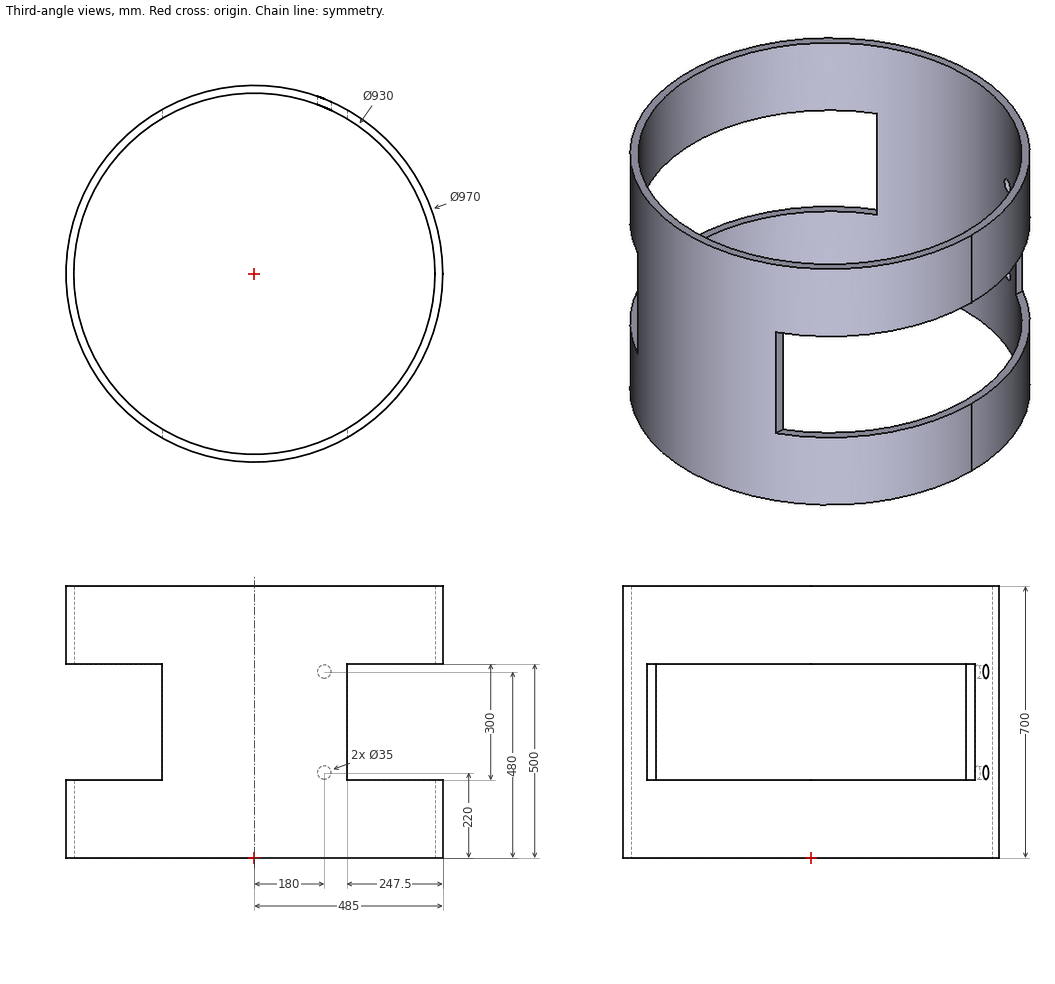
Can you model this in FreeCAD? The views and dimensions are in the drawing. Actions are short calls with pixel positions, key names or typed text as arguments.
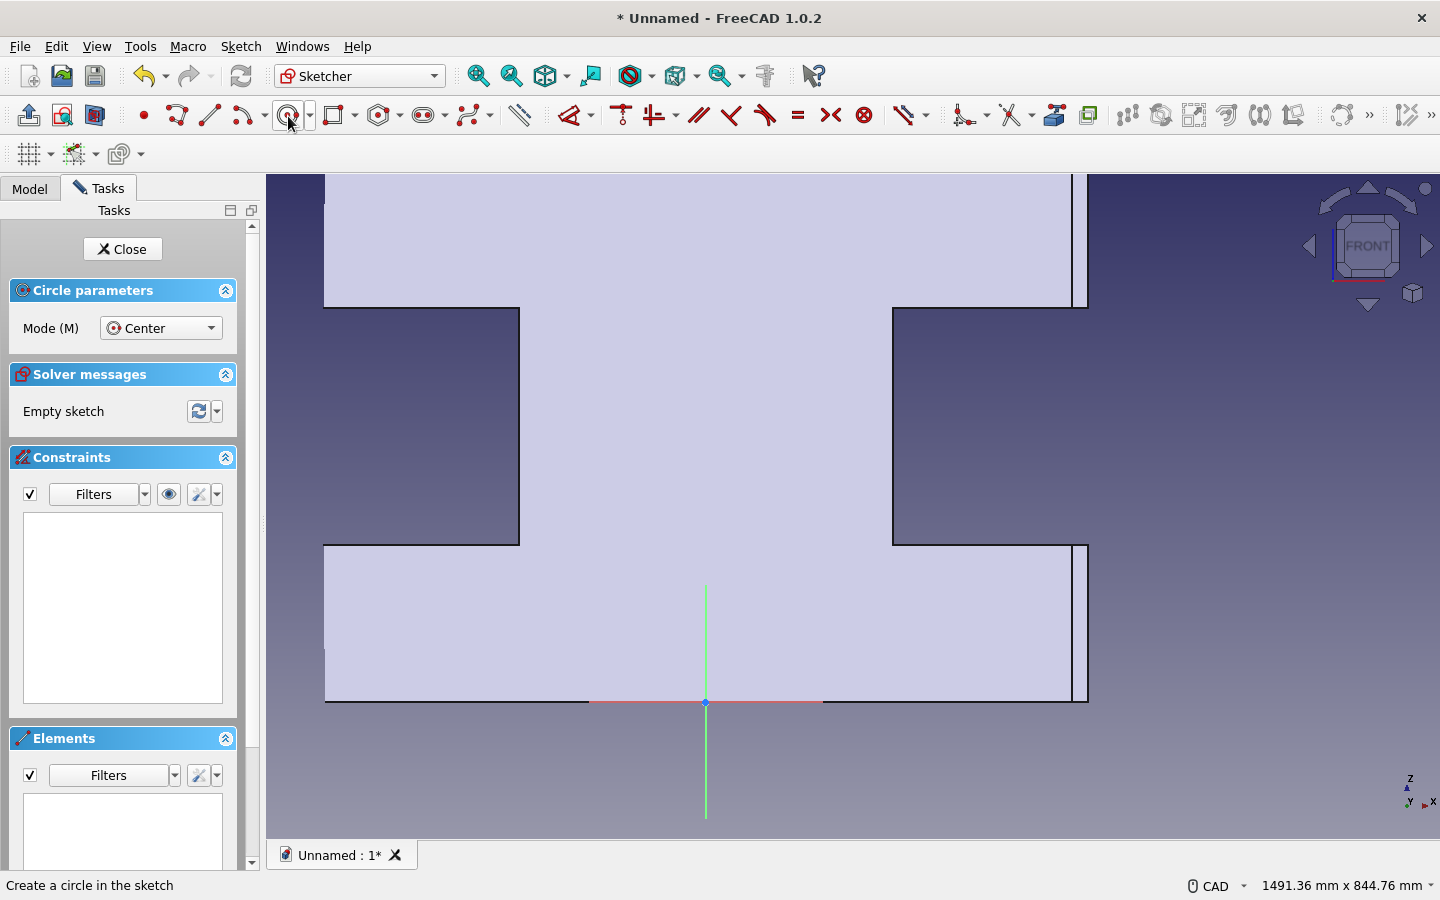
scroll(848, 529, up, 3)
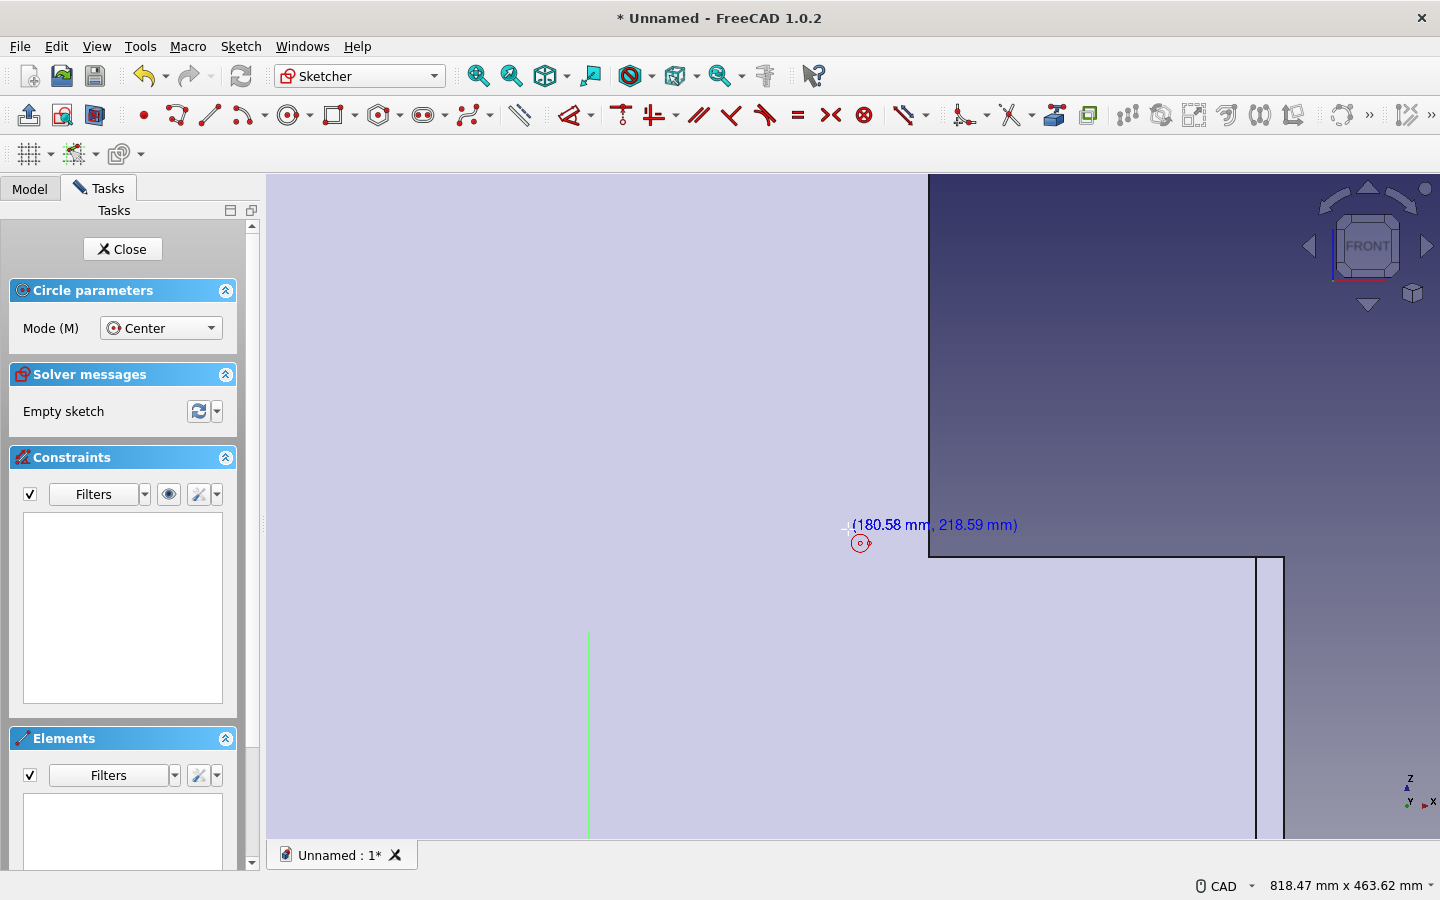
click(847, 528)
click(865, 511)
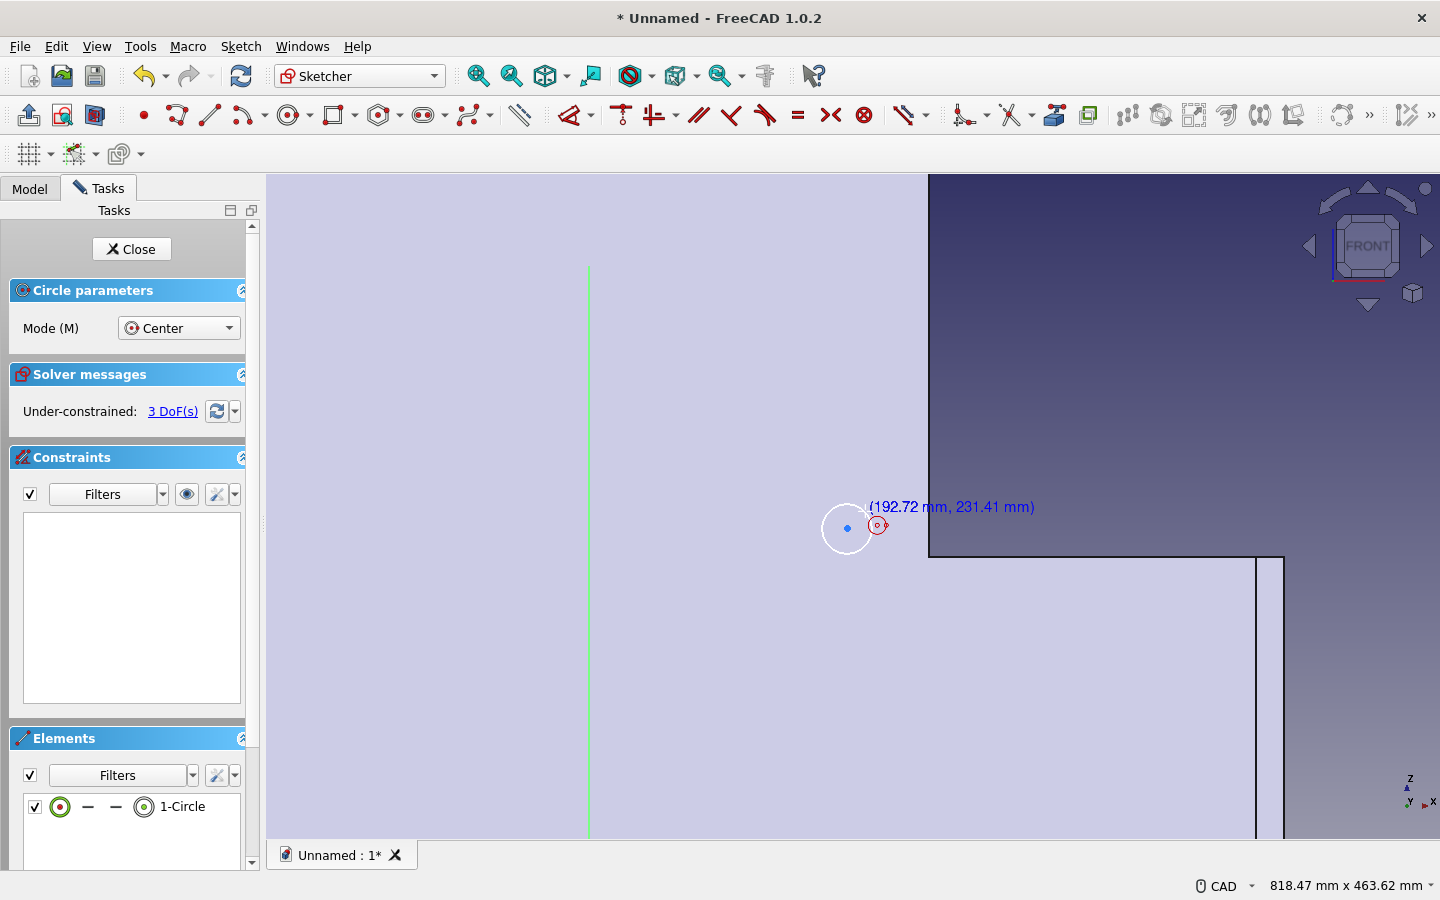
scroll(851, 530, down, 3)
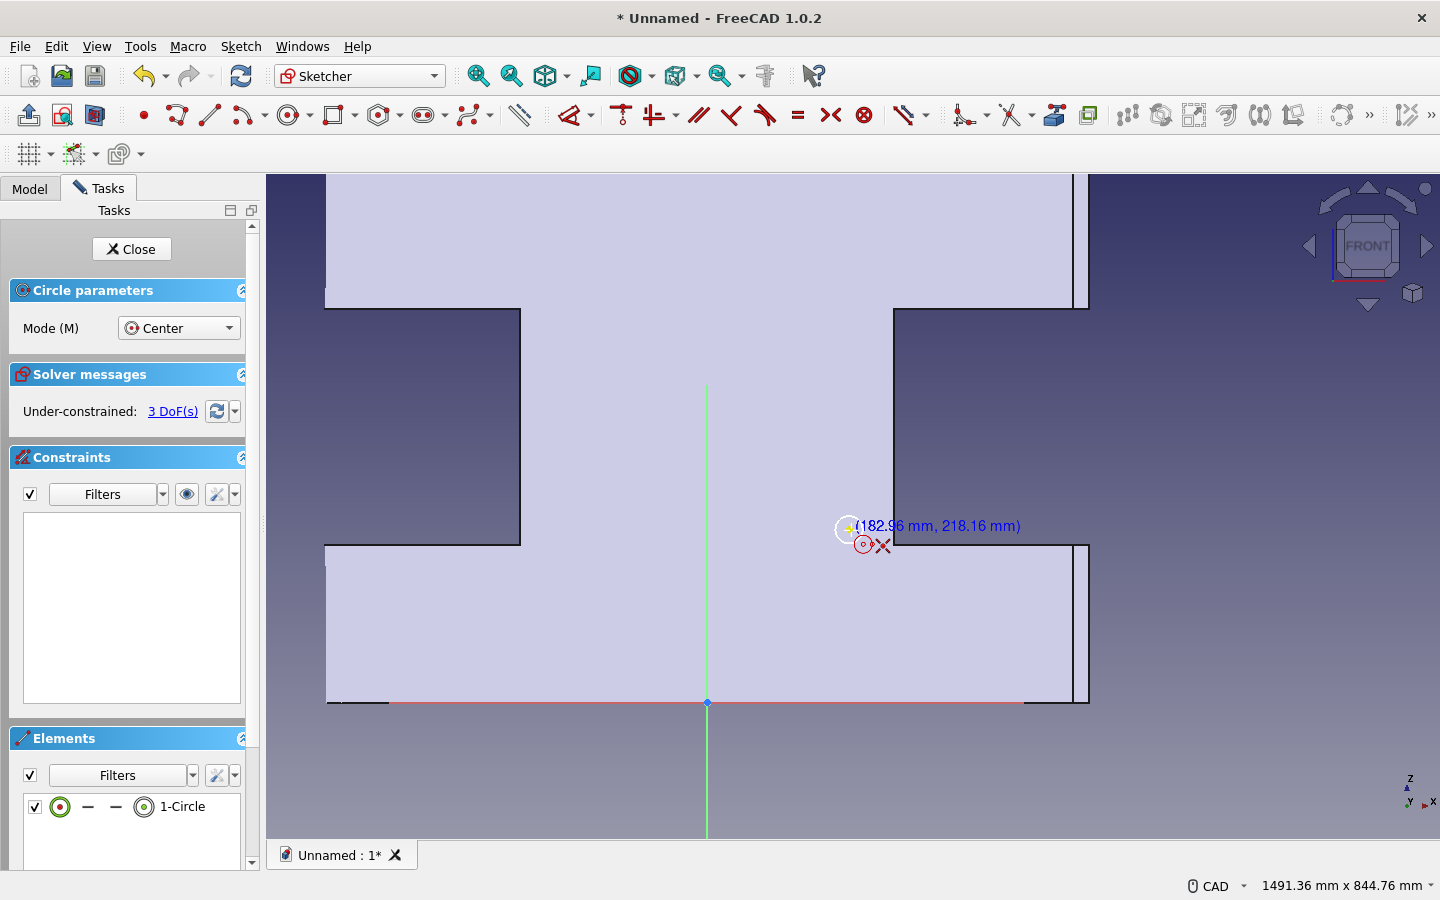
scroll(849, 325, up, 3)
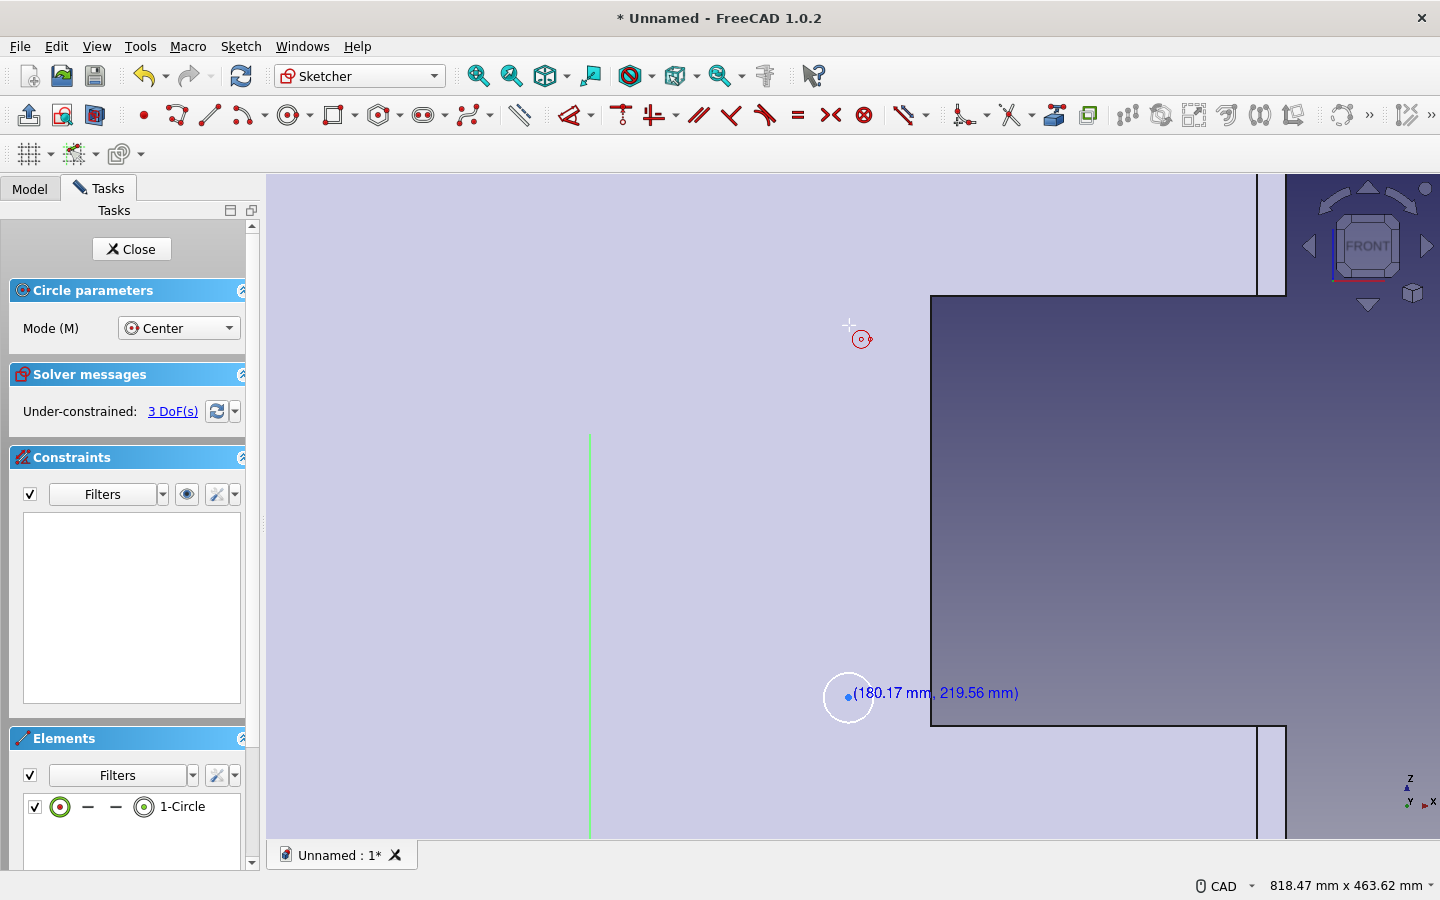
click(848, 324)
click(866, 306)
key(Escape)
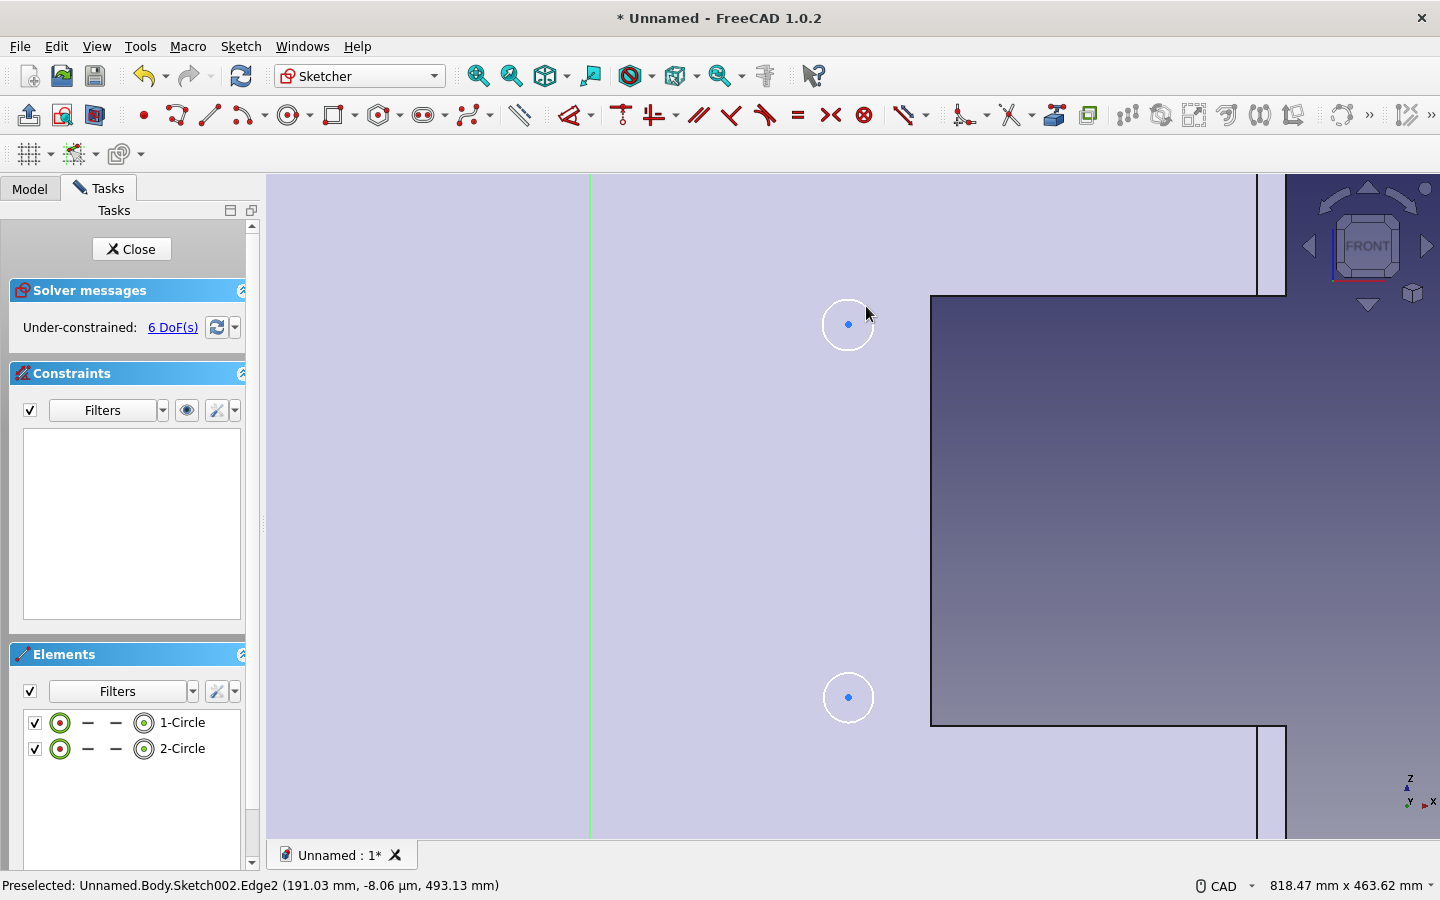
click(866, 680)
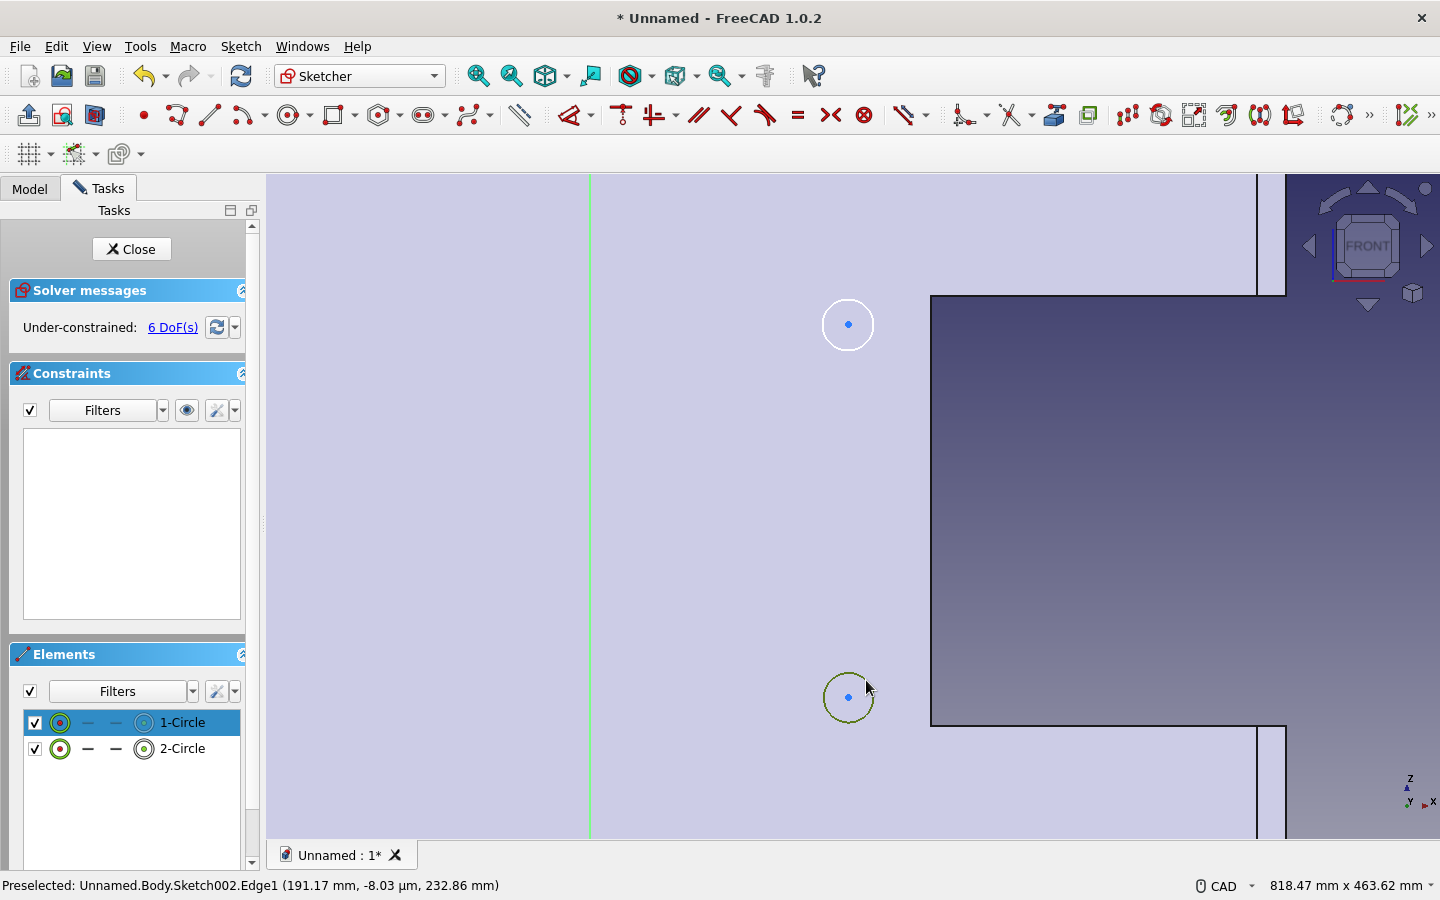
click(866, 307)